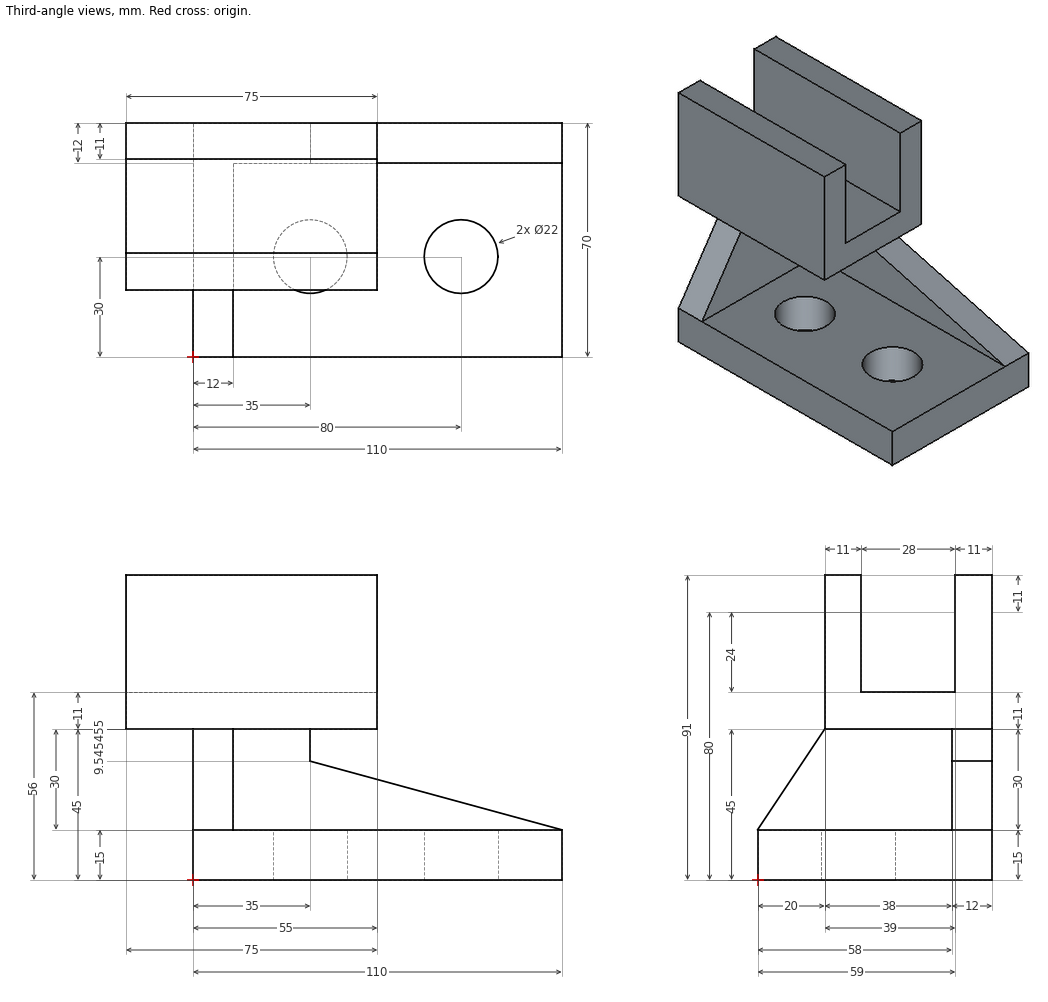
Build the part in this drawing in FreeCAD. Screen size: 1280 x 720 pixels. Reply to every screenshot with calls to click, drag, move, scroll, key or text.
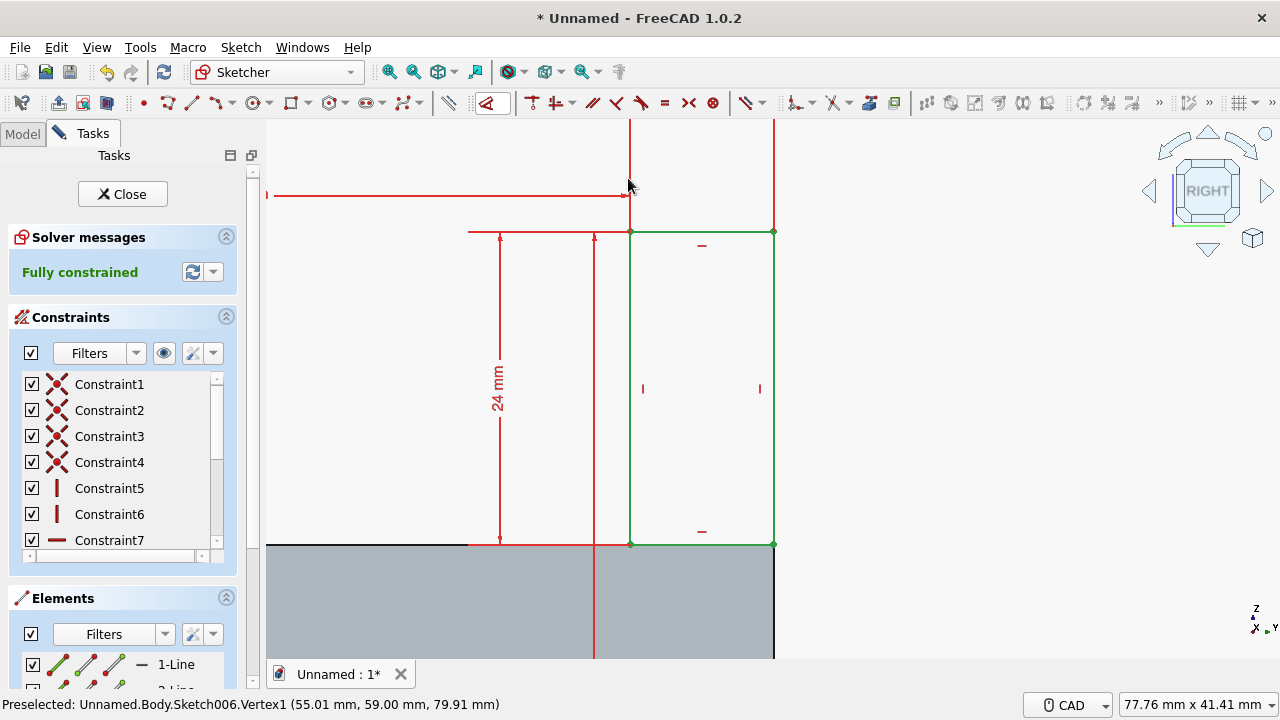
click(123, 194)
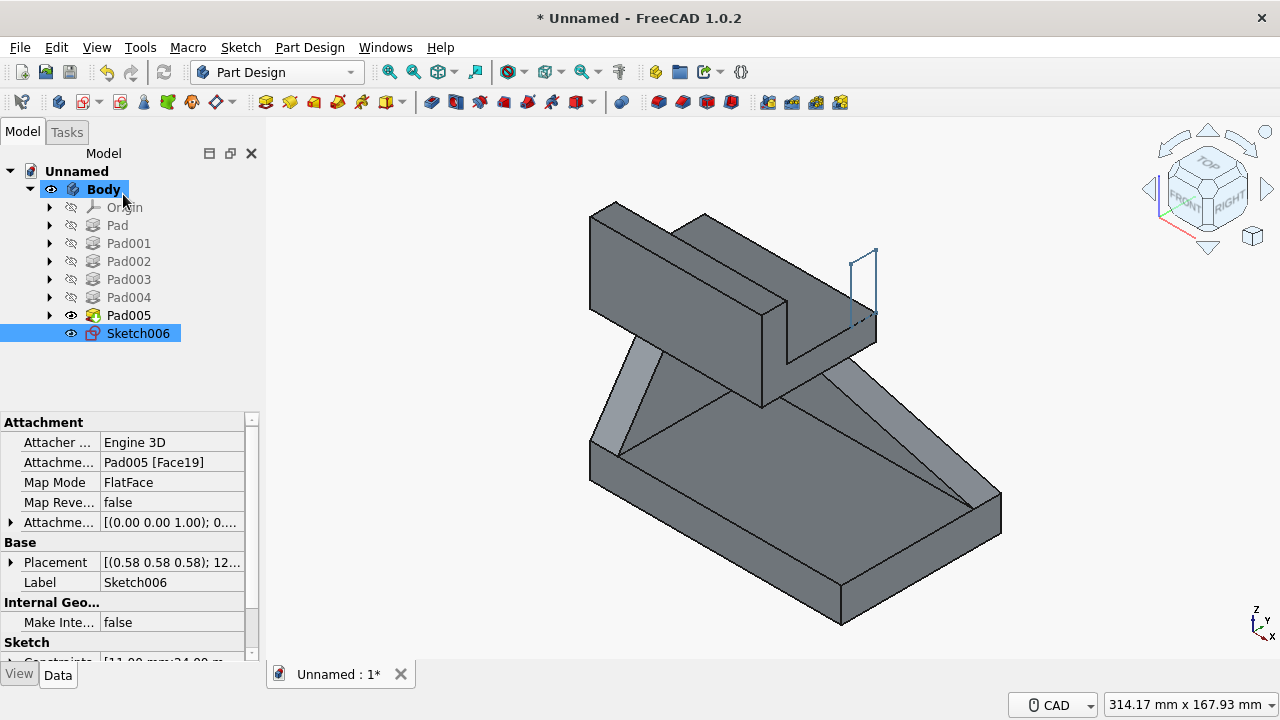
click(266, 102)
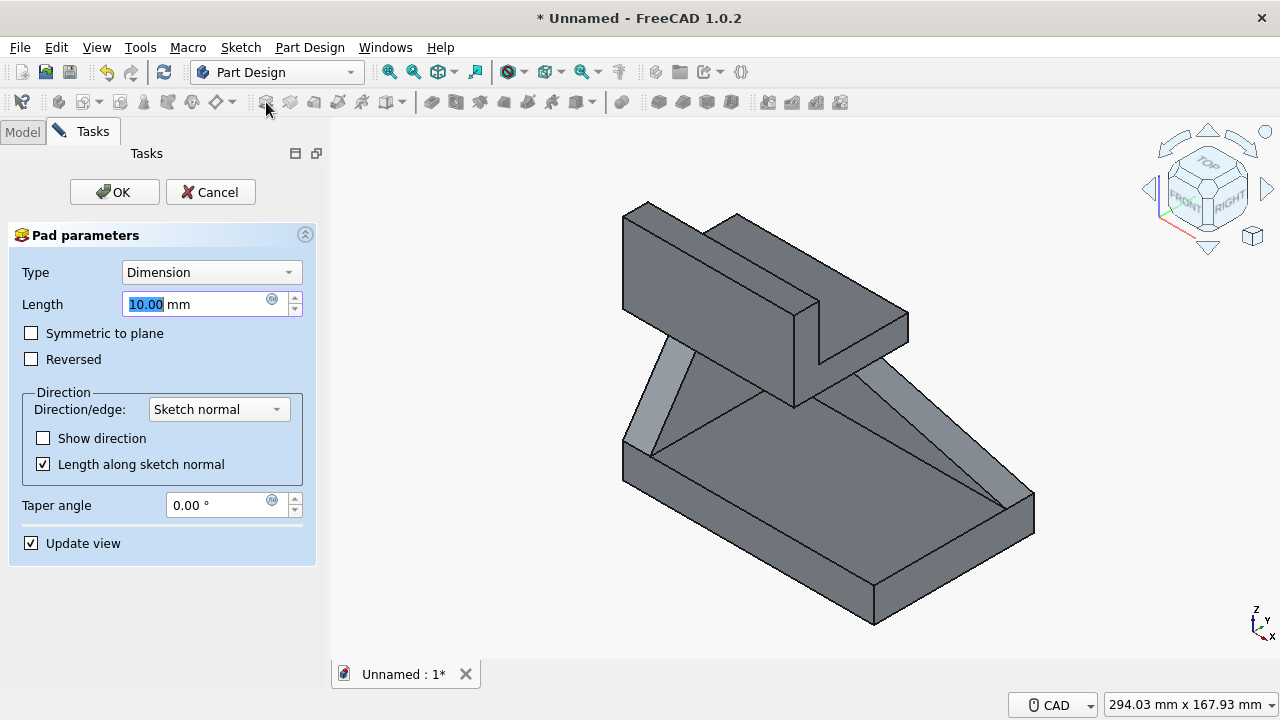
text(75)
key(Tab)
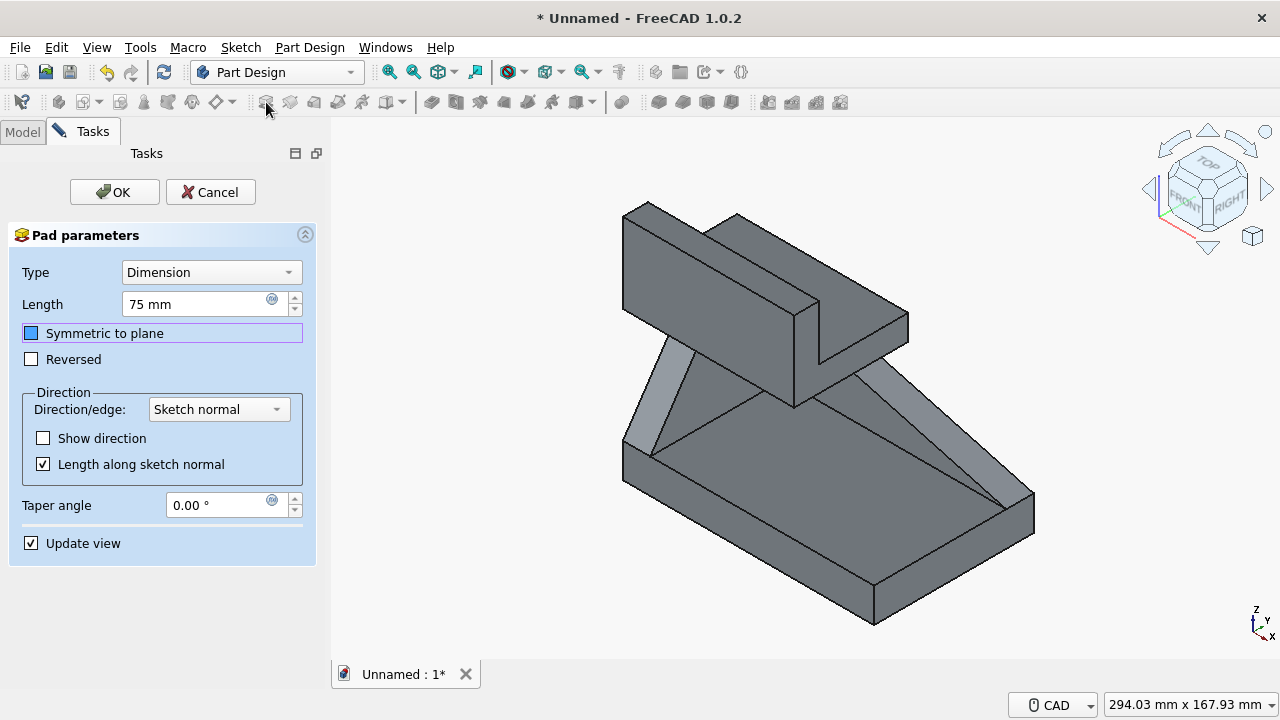
click(30, 359)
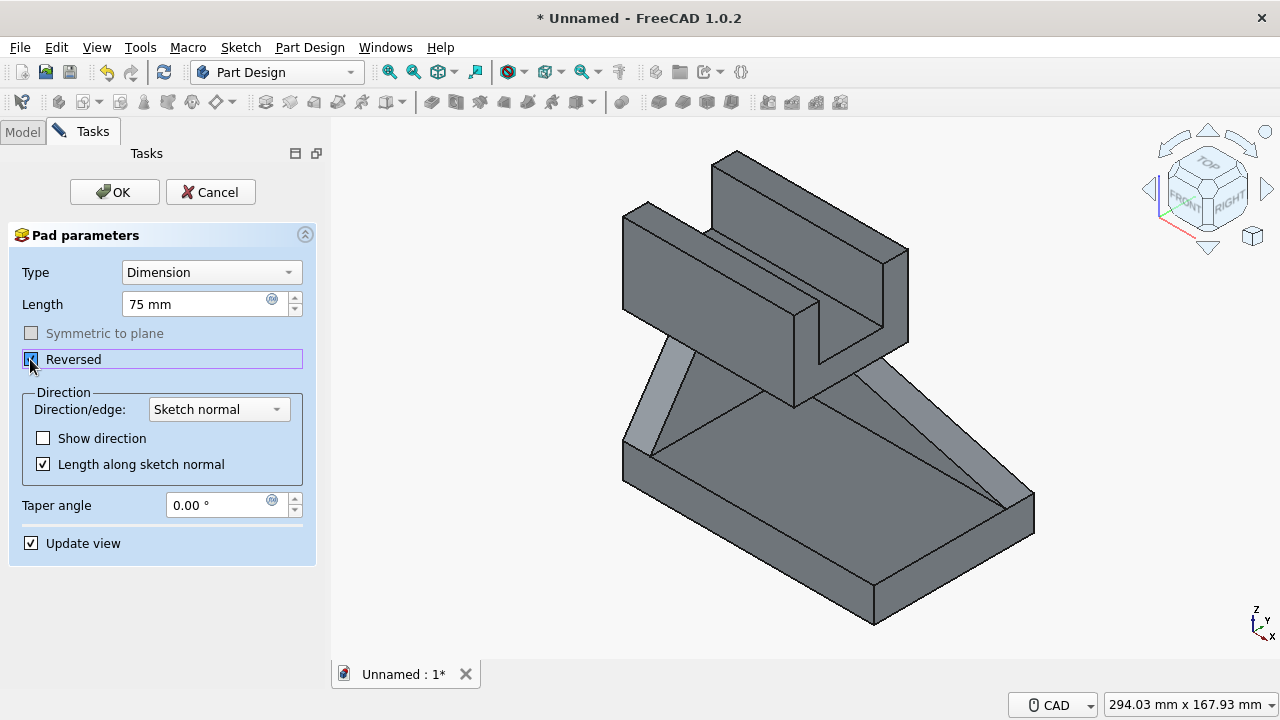
click(115, 192)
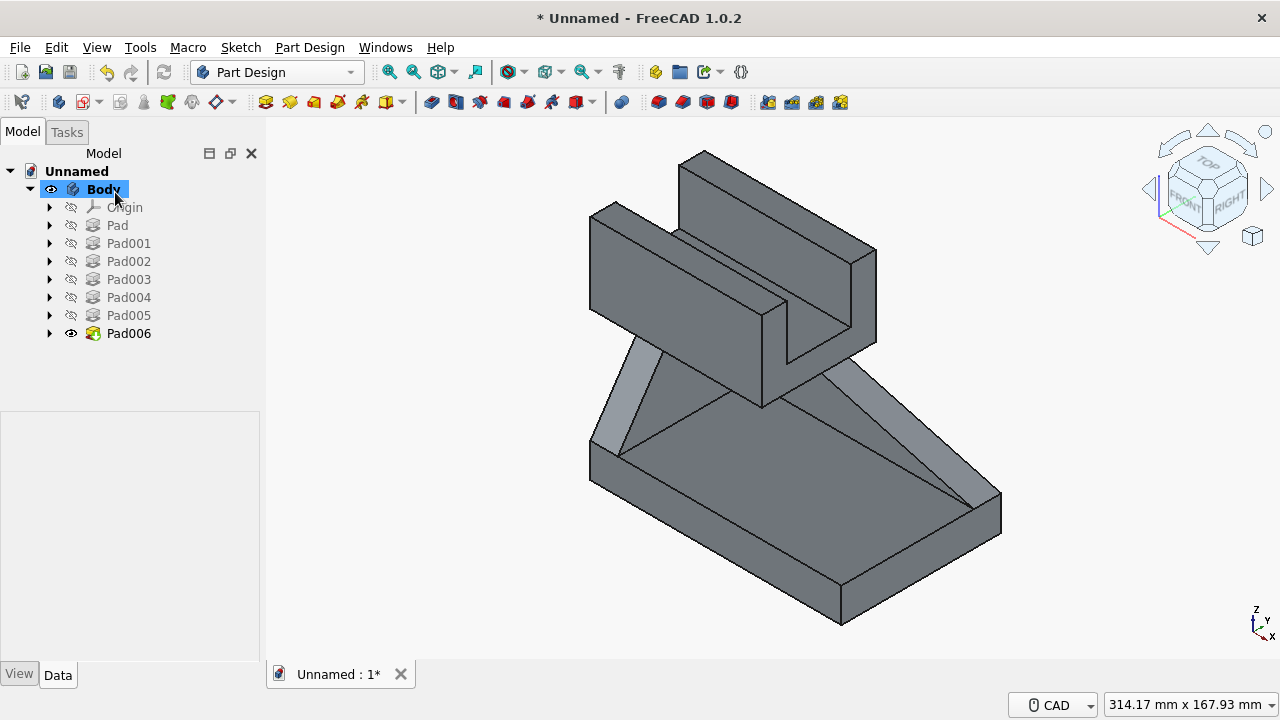
click(828, 500)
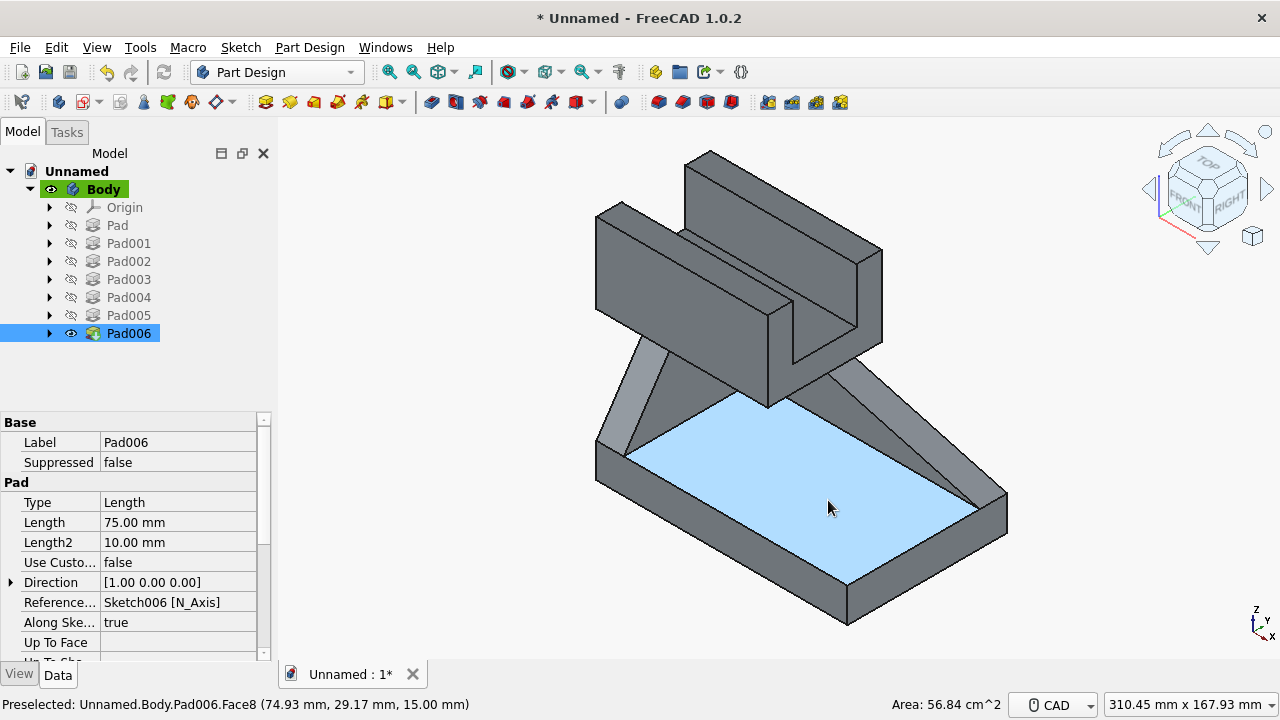
click(84, 102)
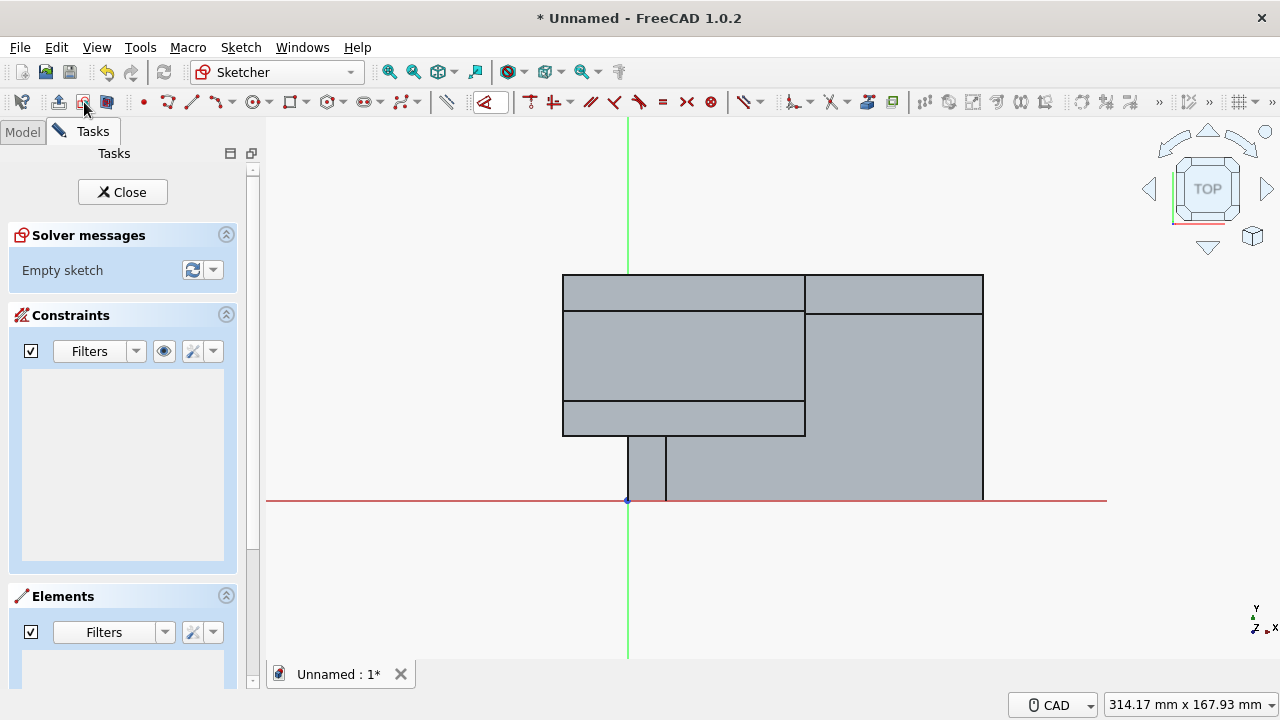
scroll(860, 492, up, 3)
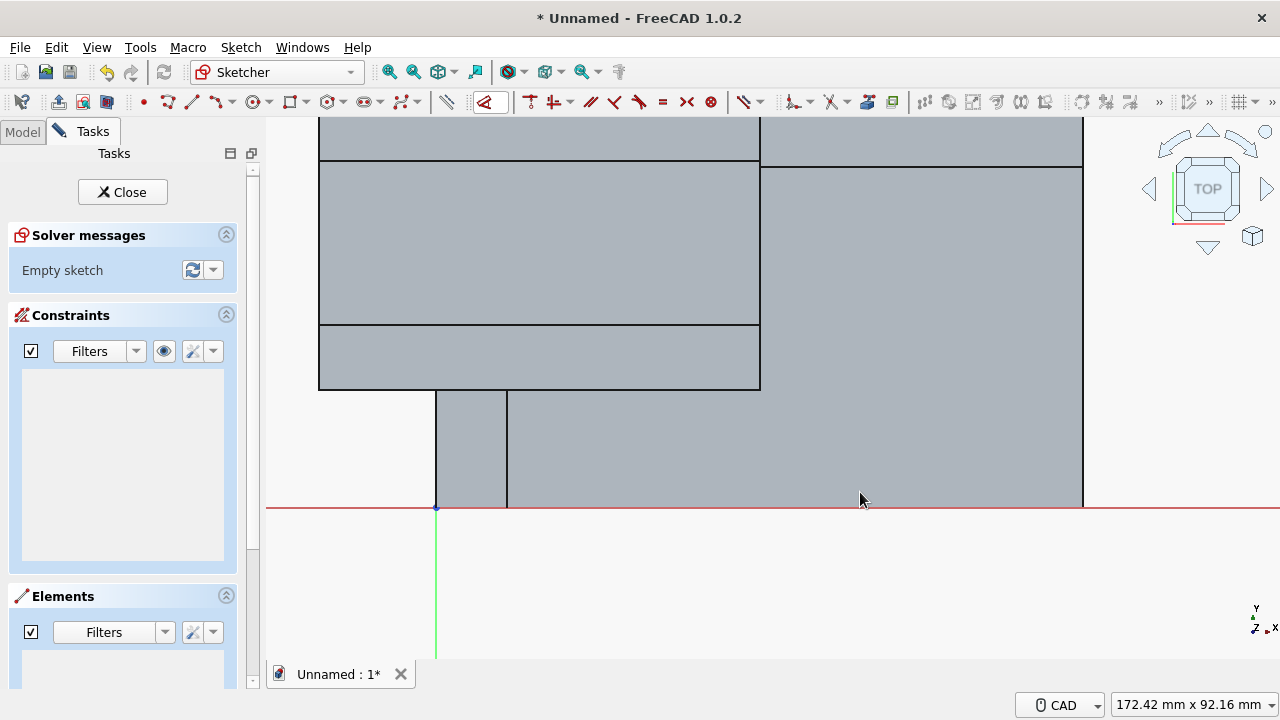
key(g)
key(c)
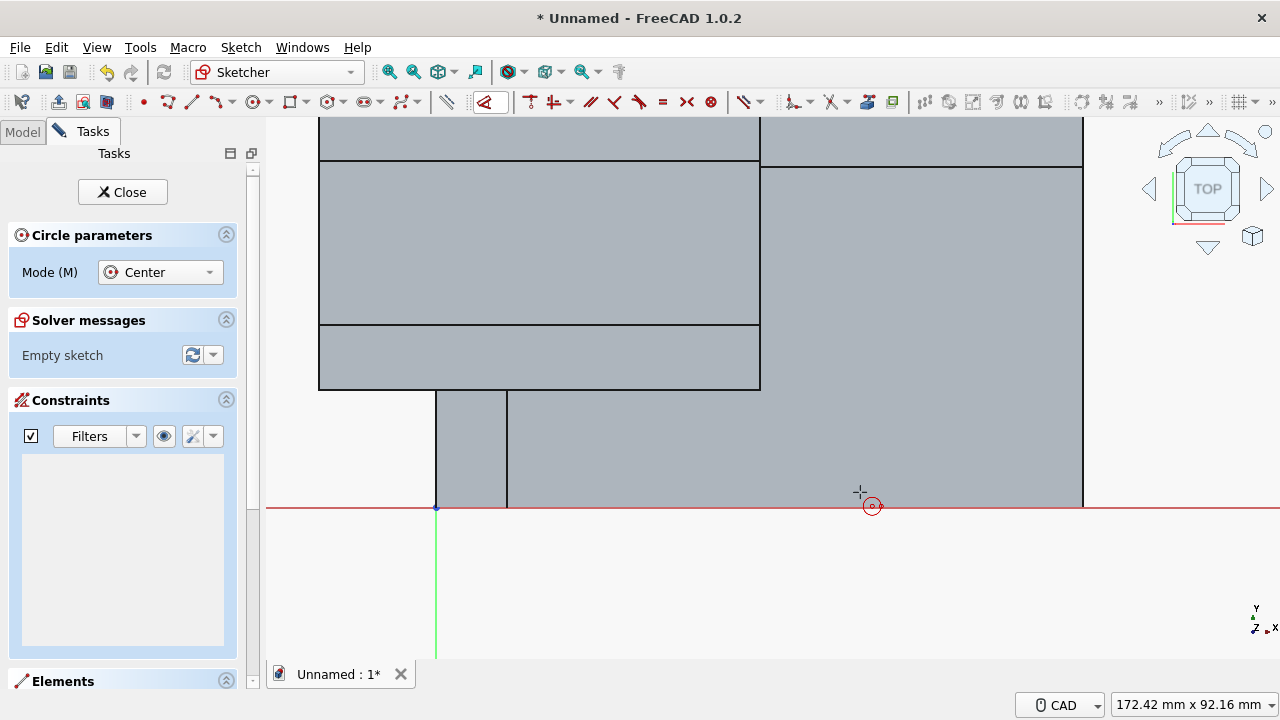
click(907, 331)
move(953, 286)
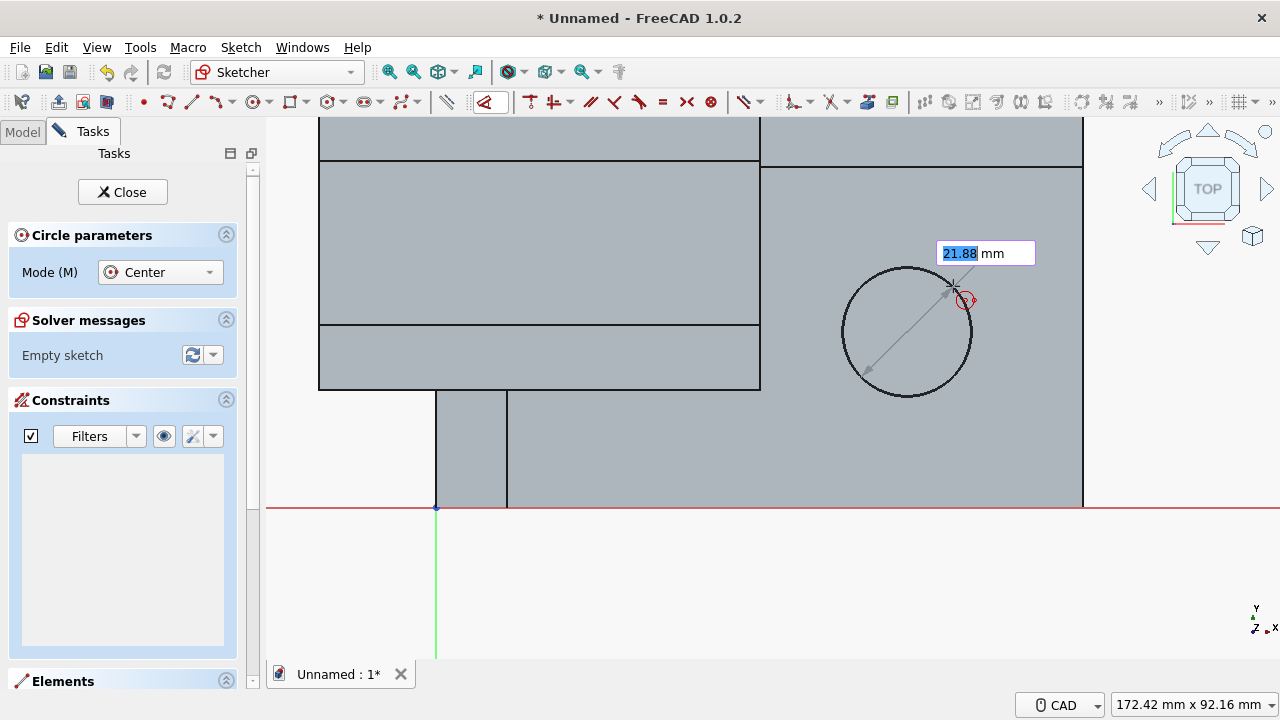
text(22)
key(Return)